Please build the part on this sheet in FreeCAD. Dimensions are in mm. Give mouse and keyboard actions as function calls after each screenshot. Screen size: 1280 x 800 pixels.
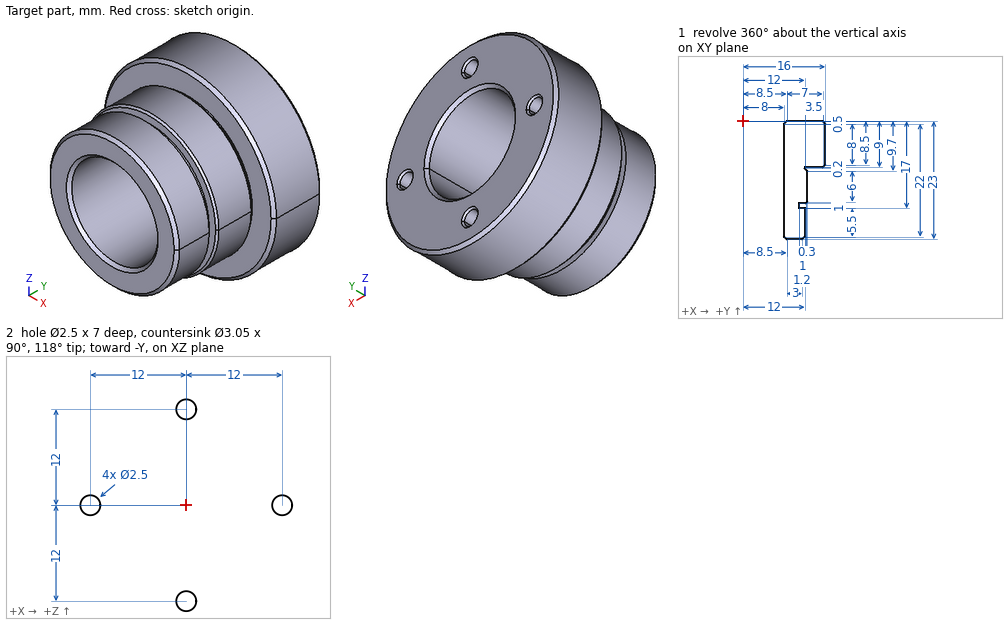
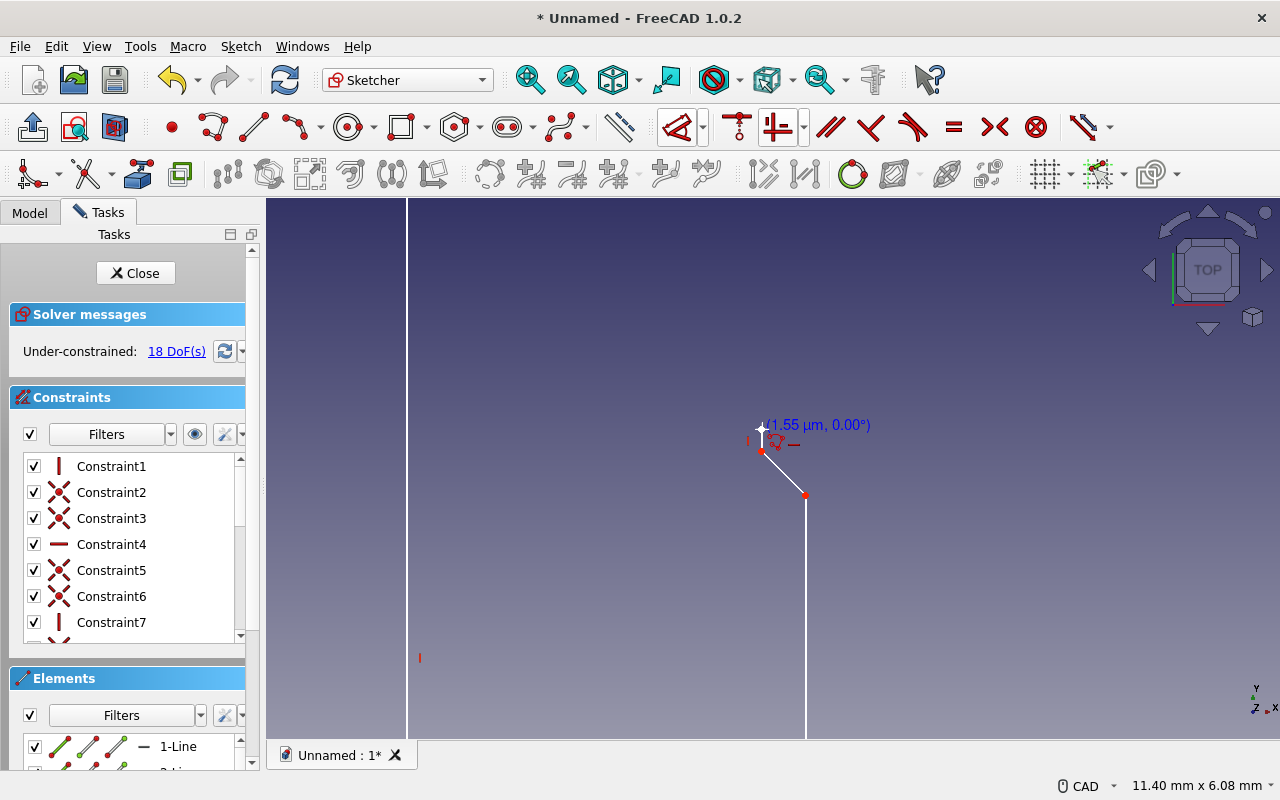
scroll(764, 432, down, 9)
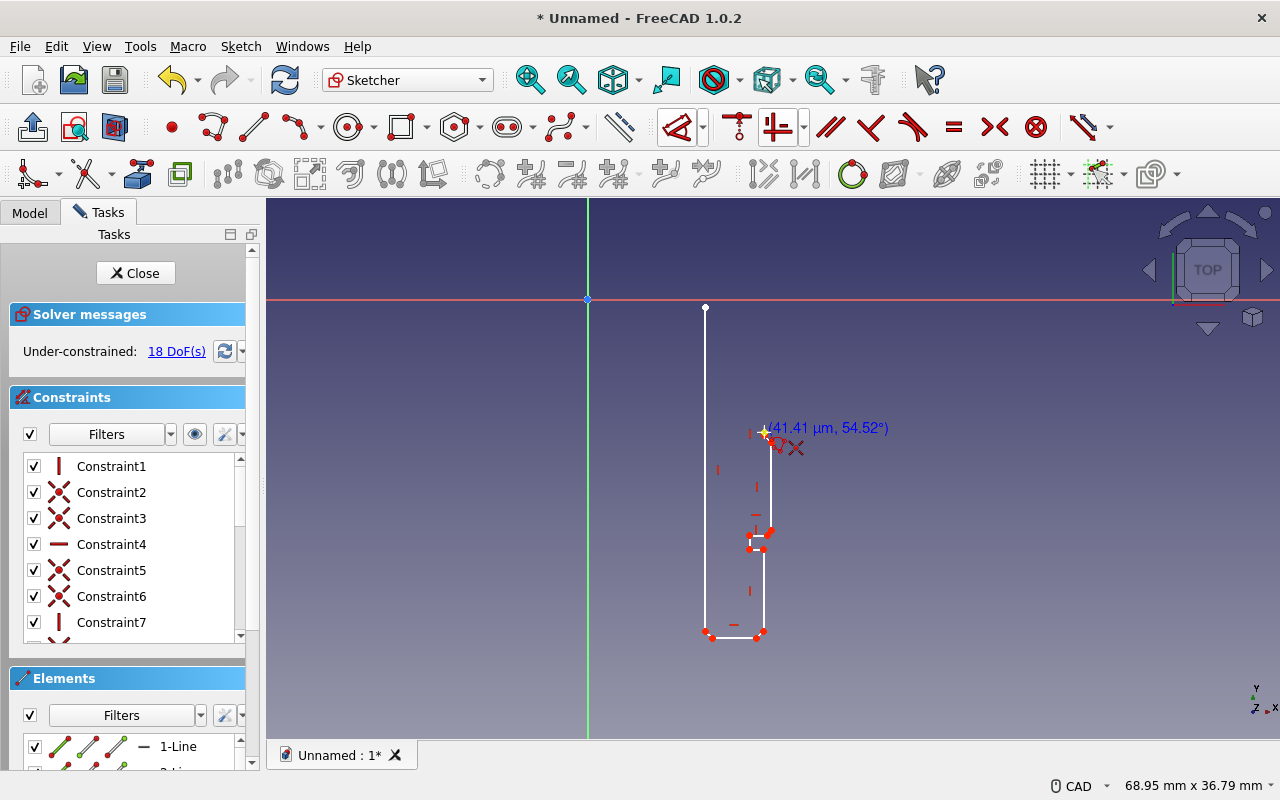
click(815, 432)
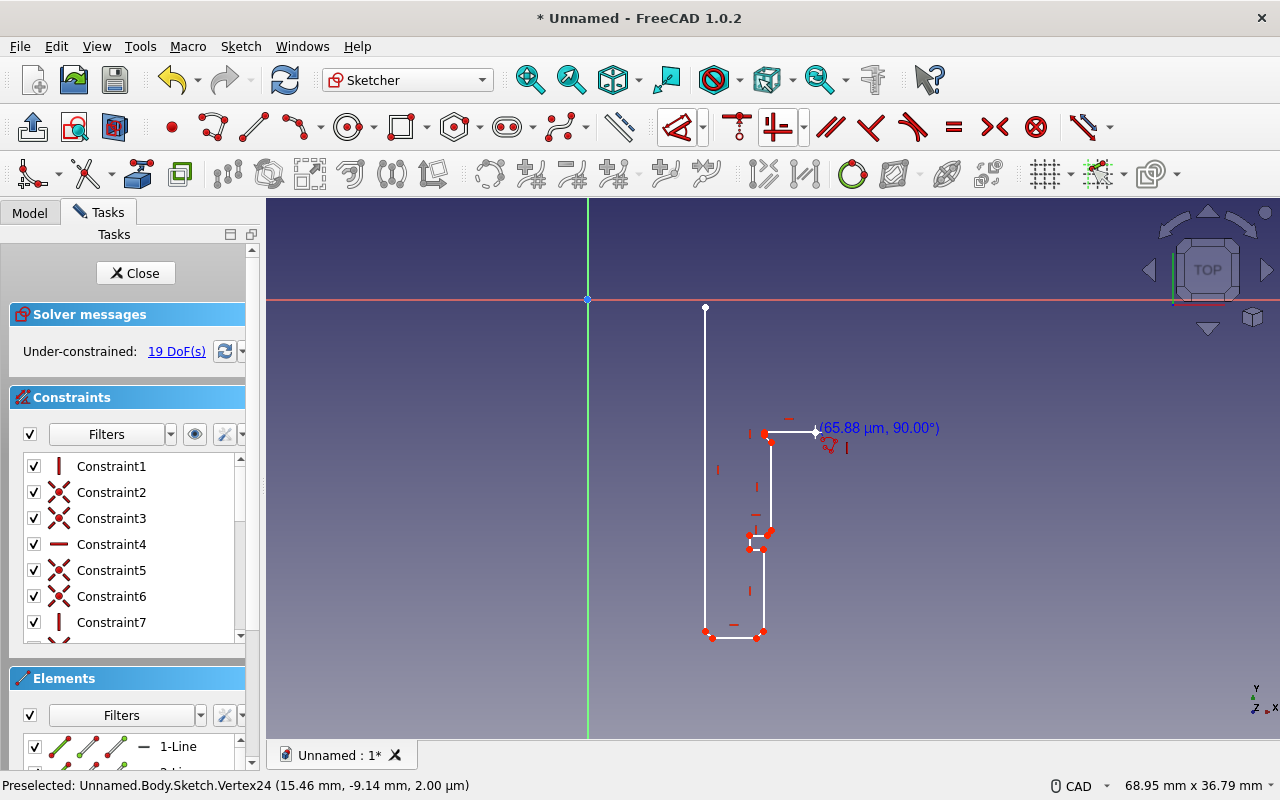
scroll(823, 425, up, 3)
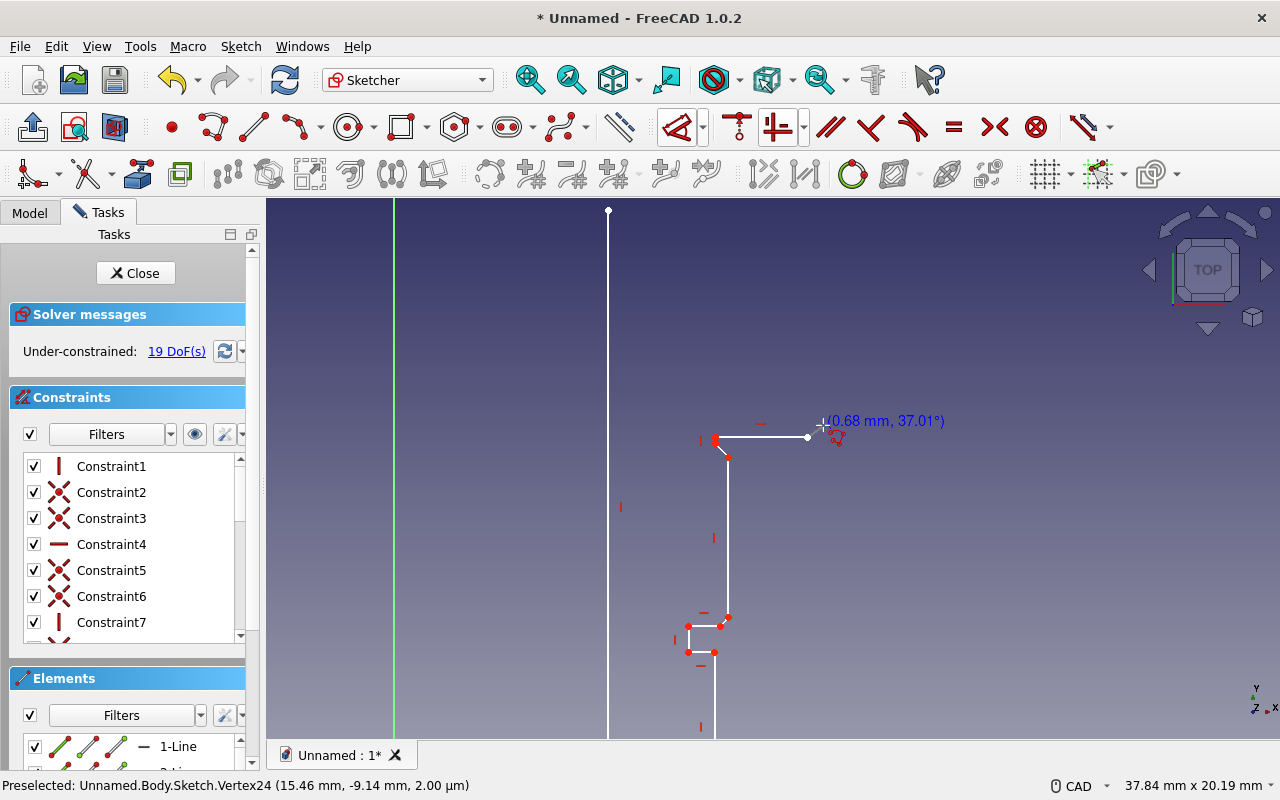
click(822, 424)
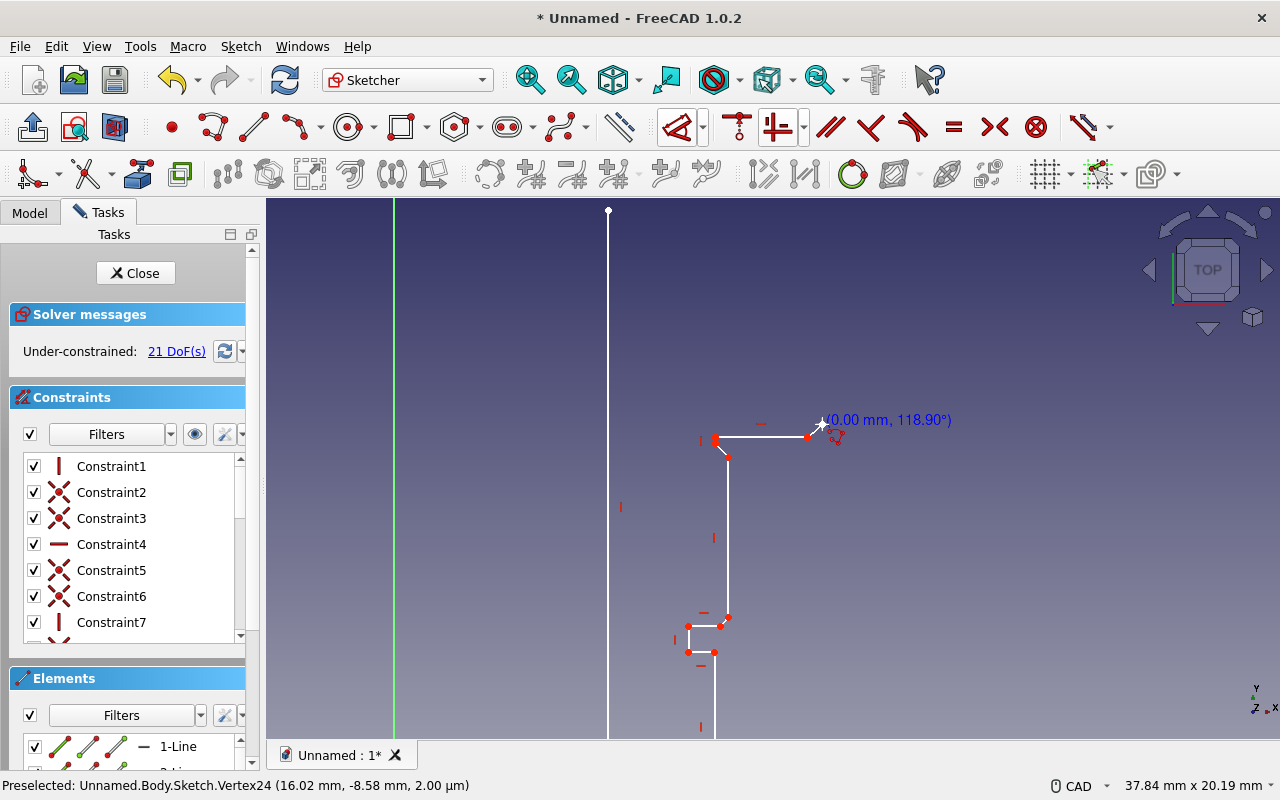
scroll(822, 425, down, 3)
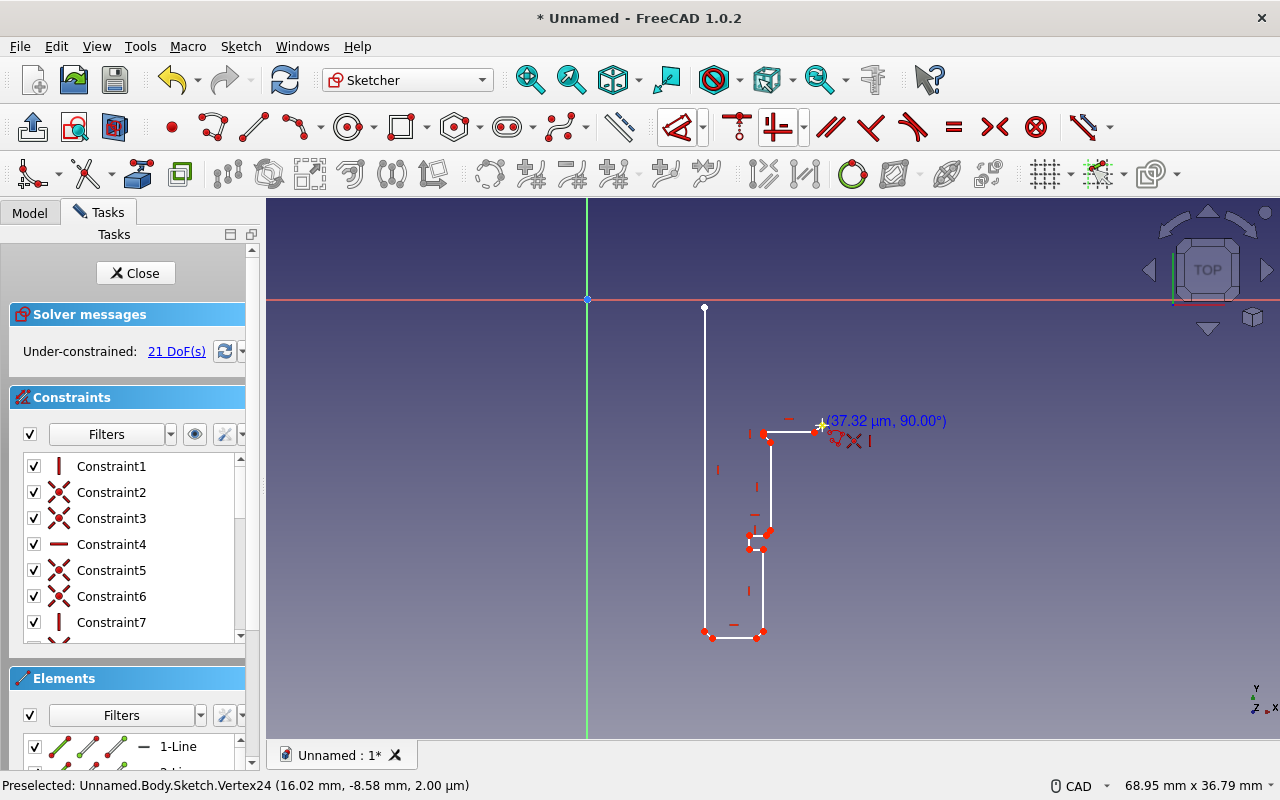
scroll(822, 307, up, 4)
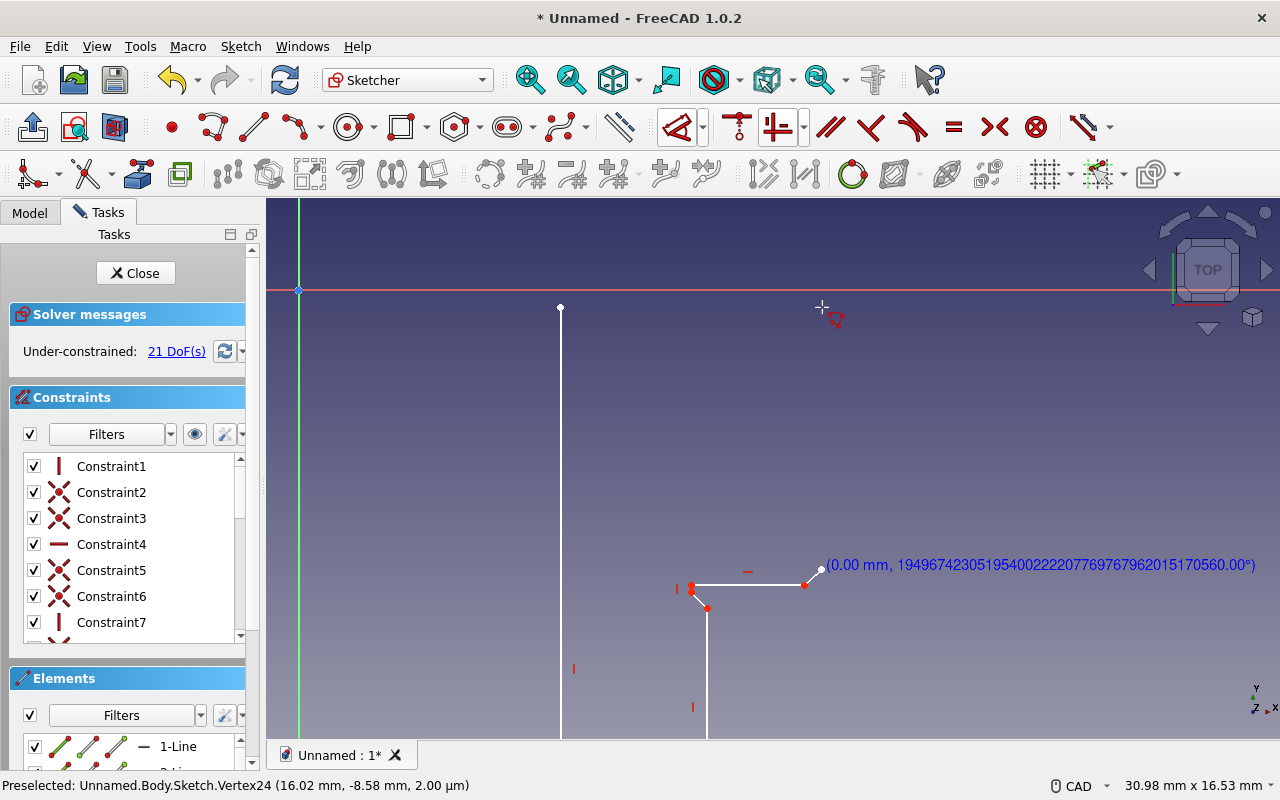
click(822, 307)
click(806, 290)
click(577, 299)
click(561, 308)
key(Escape)
key(Escape)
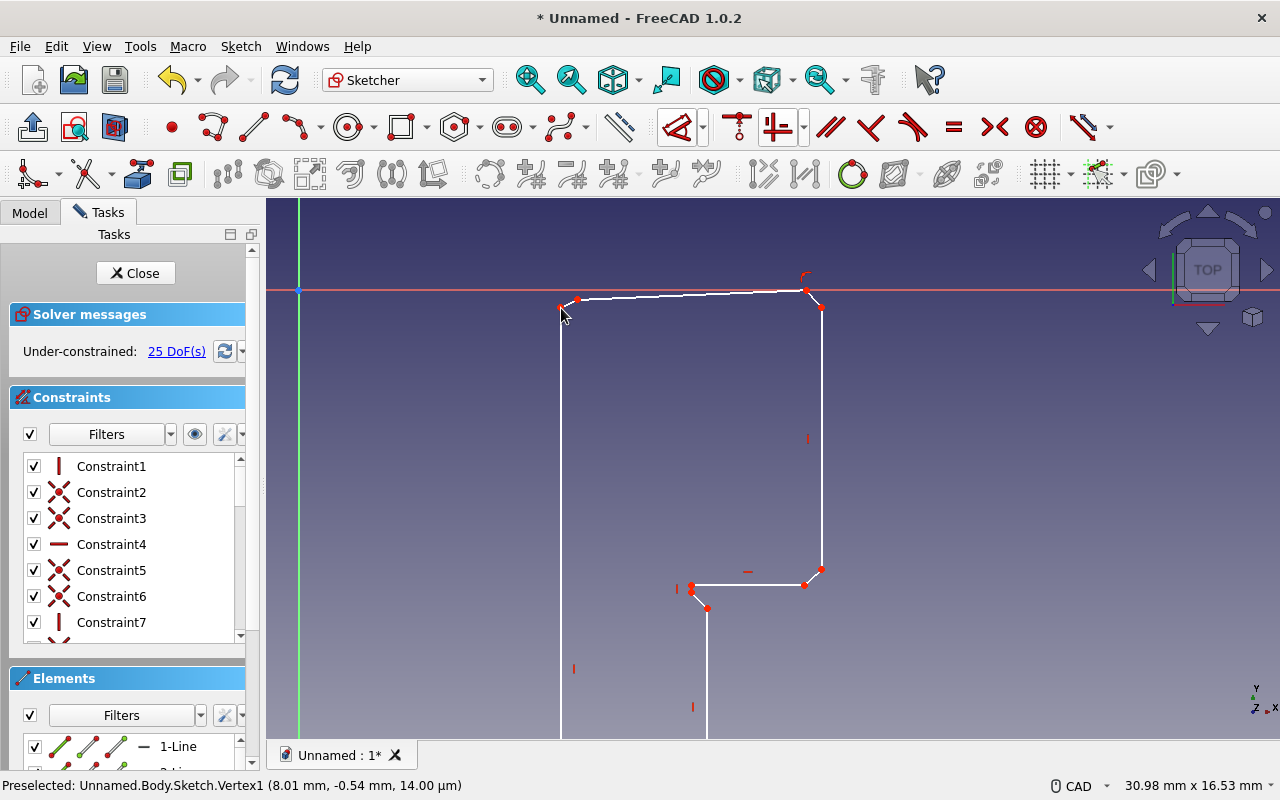
click(737, 293)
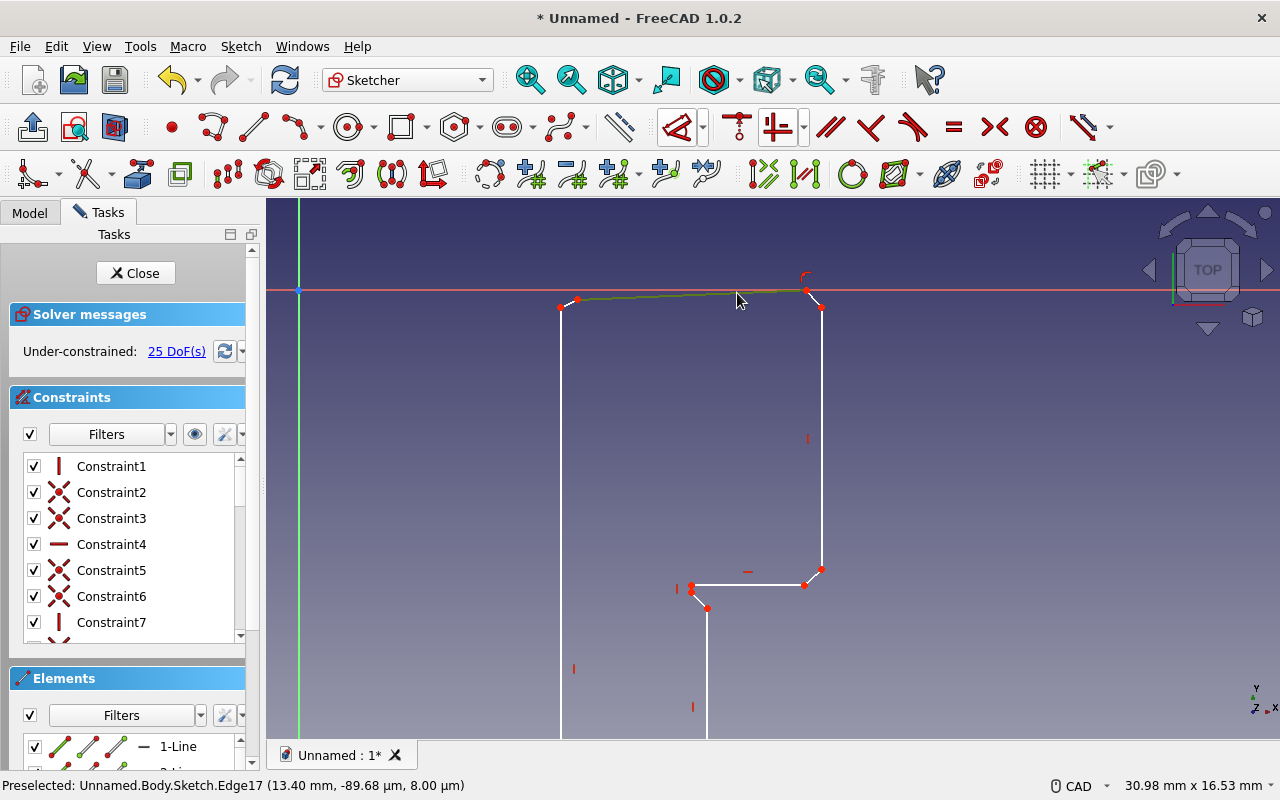
key(h)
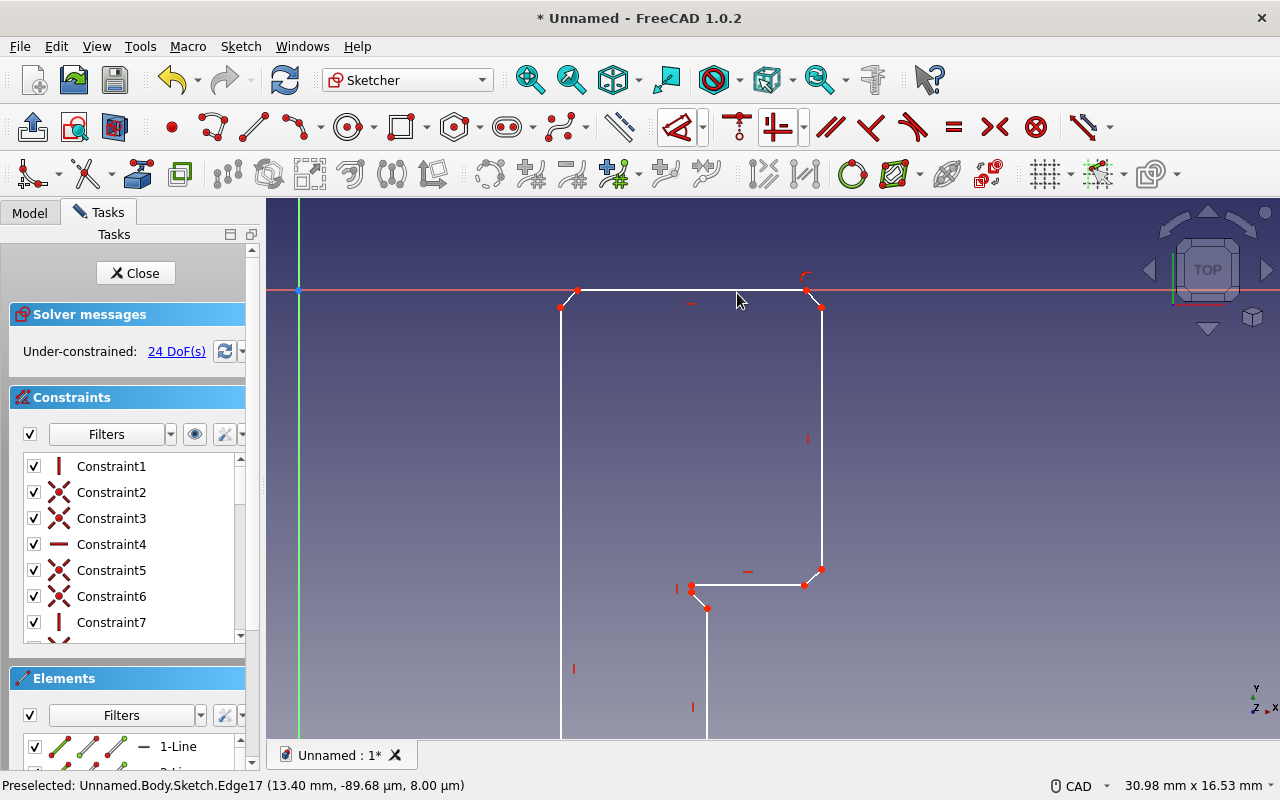
key(d)